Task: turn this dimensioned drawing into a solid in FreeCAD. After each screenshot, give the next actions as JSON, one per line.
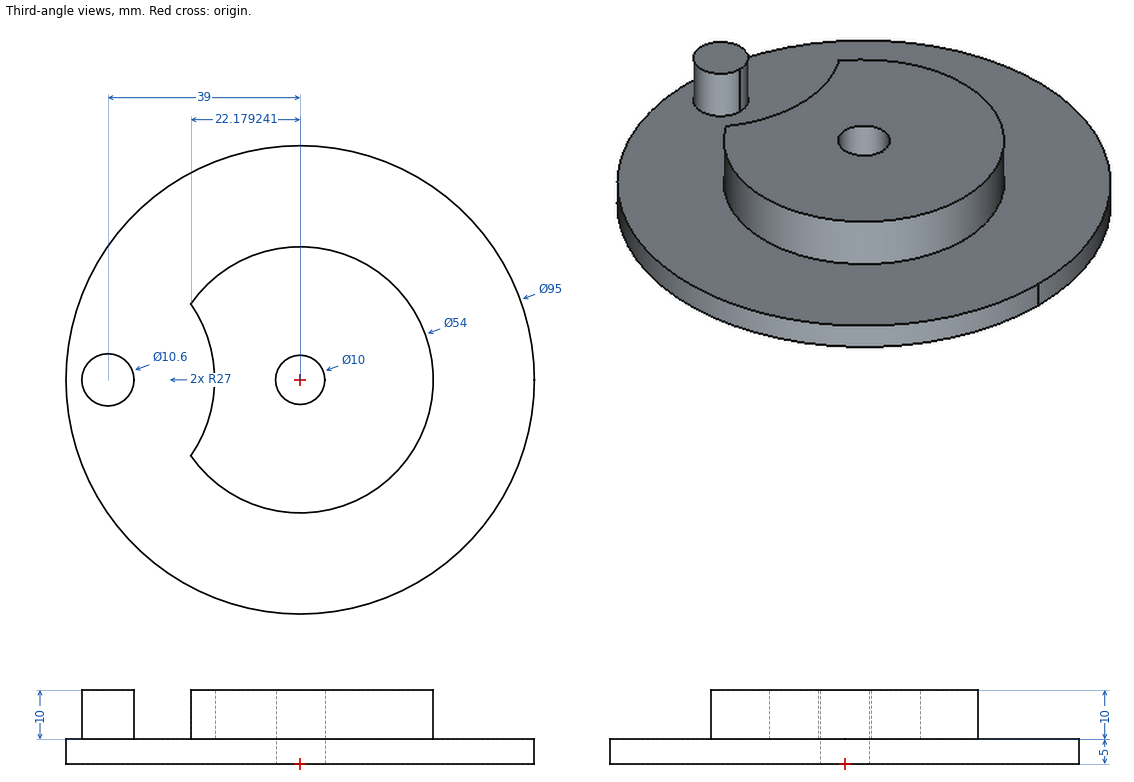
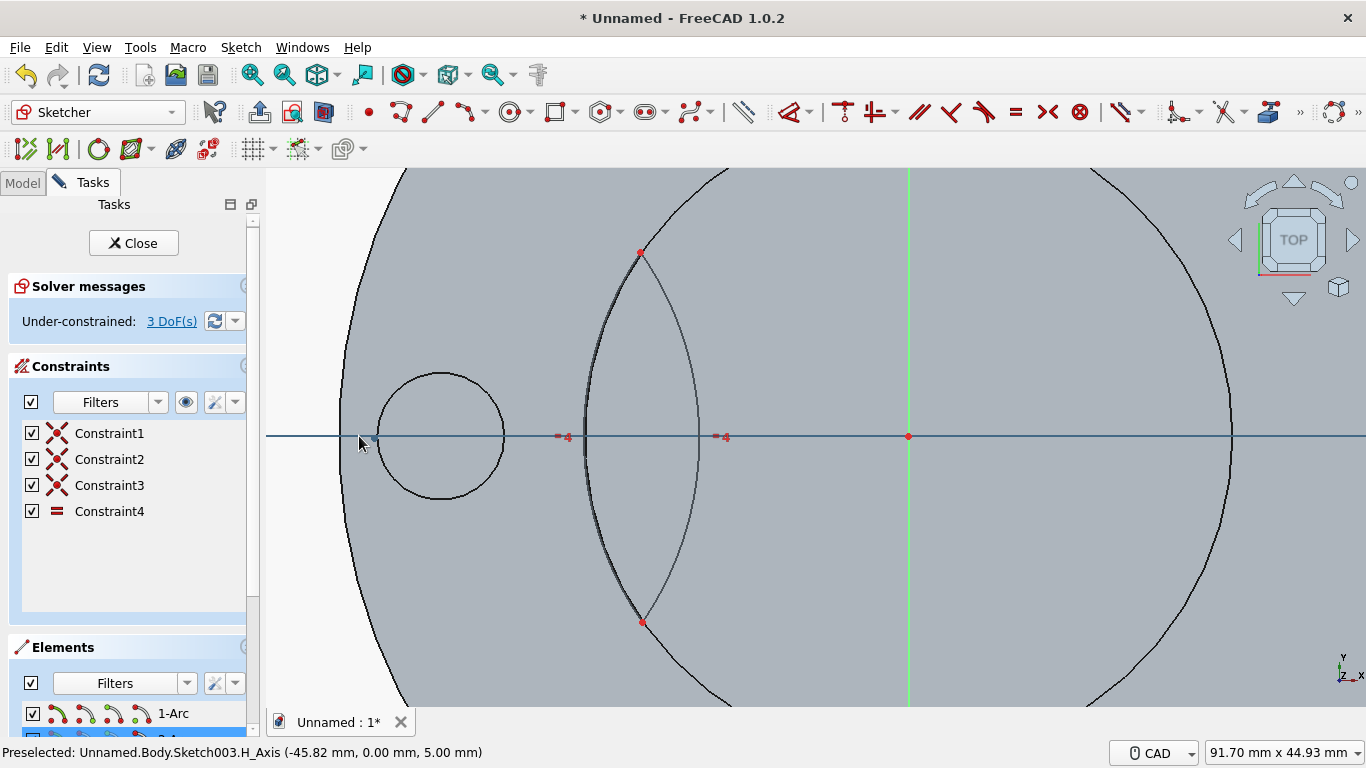
{"action": "key", "text": "c"}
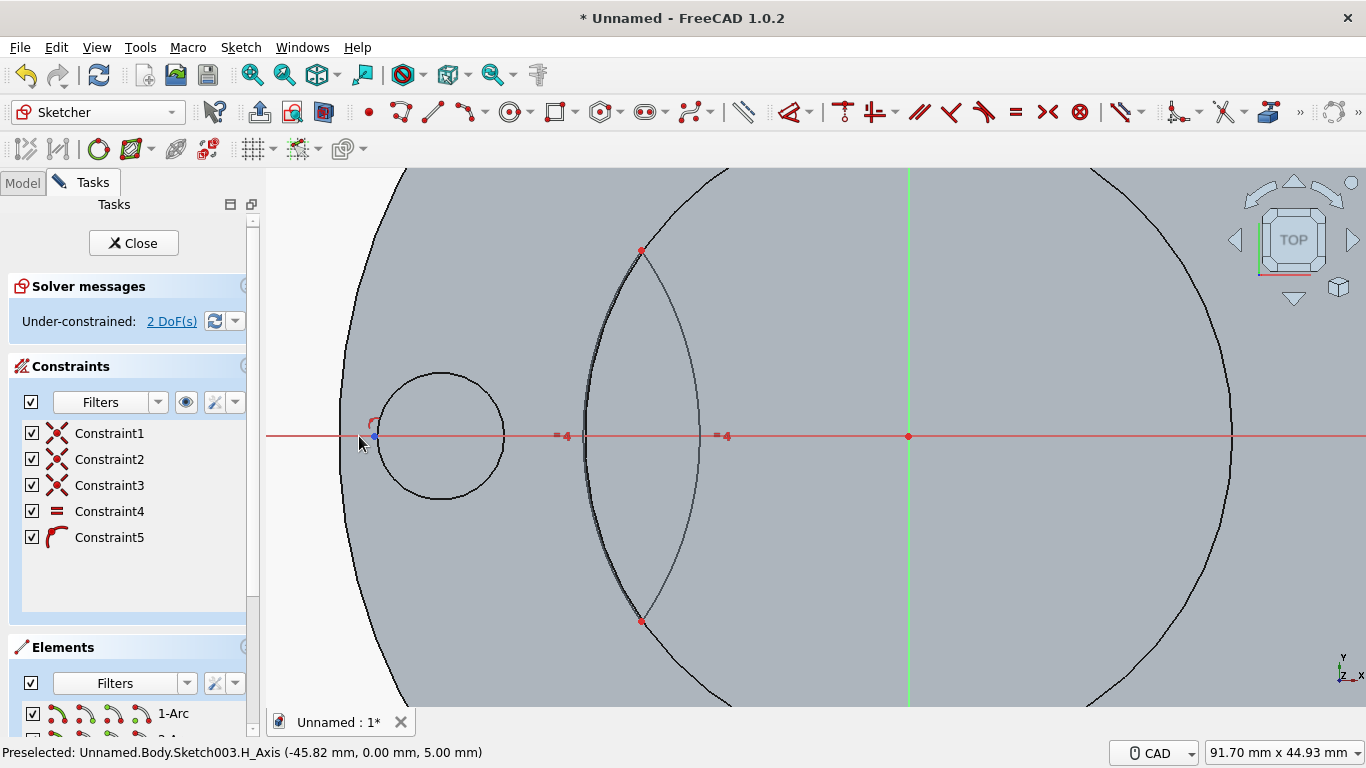
{"action": "key", "text": "d"}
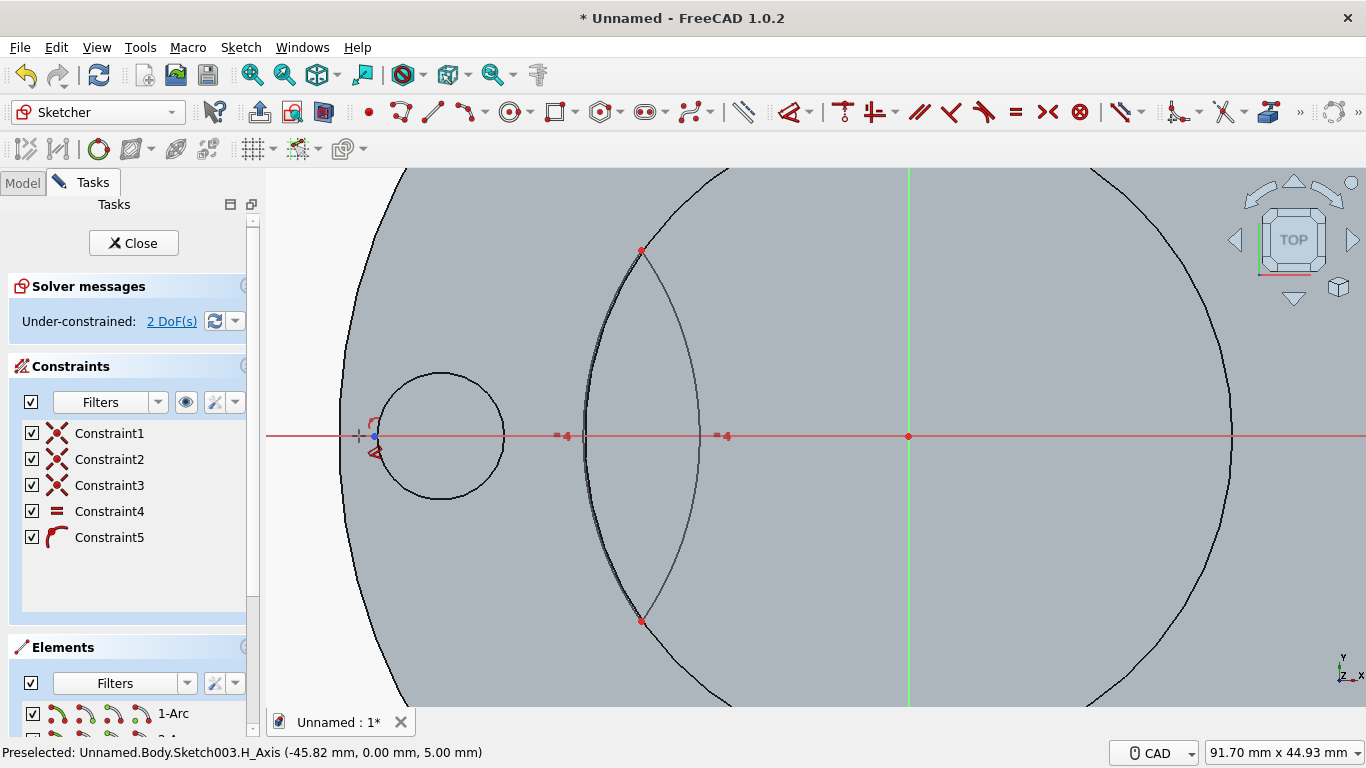
{"action": "left_click", "coordinate": [593, 358]}
{"action": "left_click", "coordinate": [562, 350]}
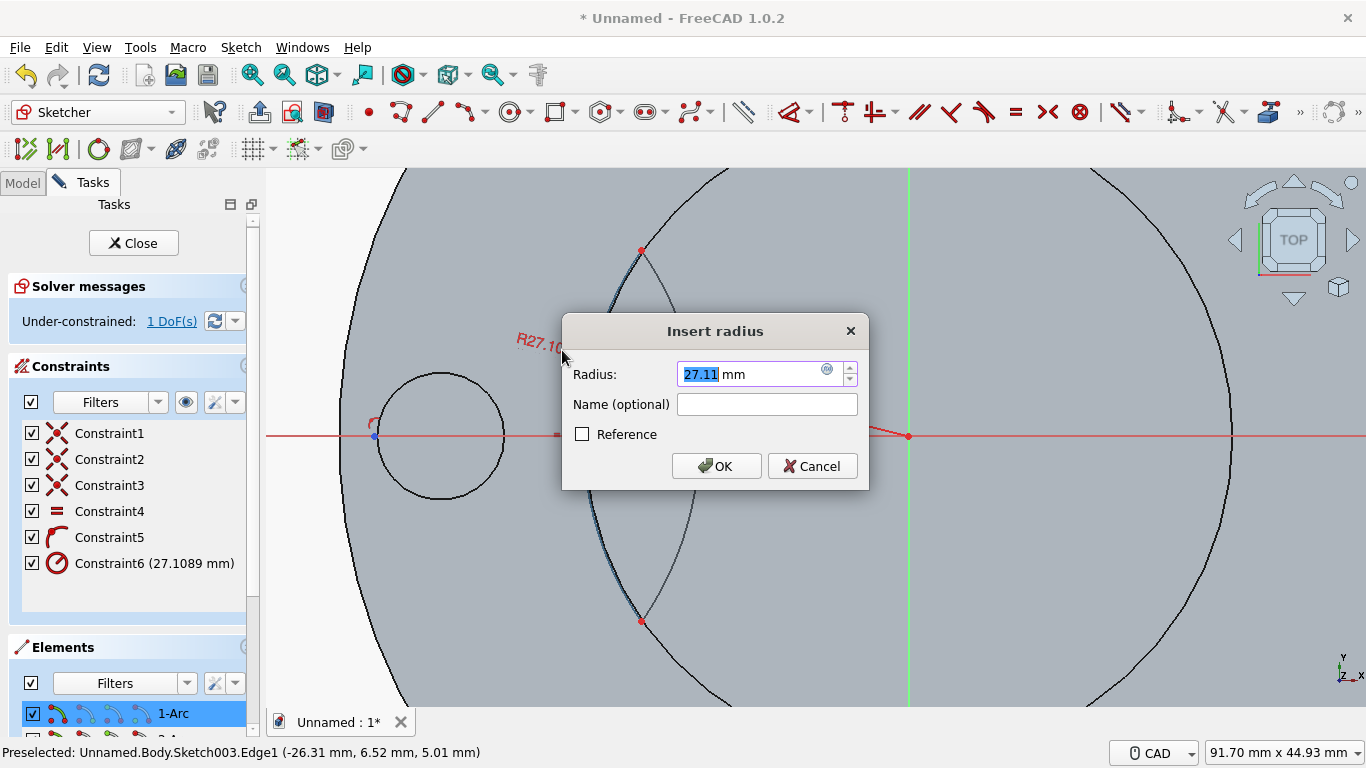
{"action": "type", "text": "27"}
{"action": "key", "text": "Return"}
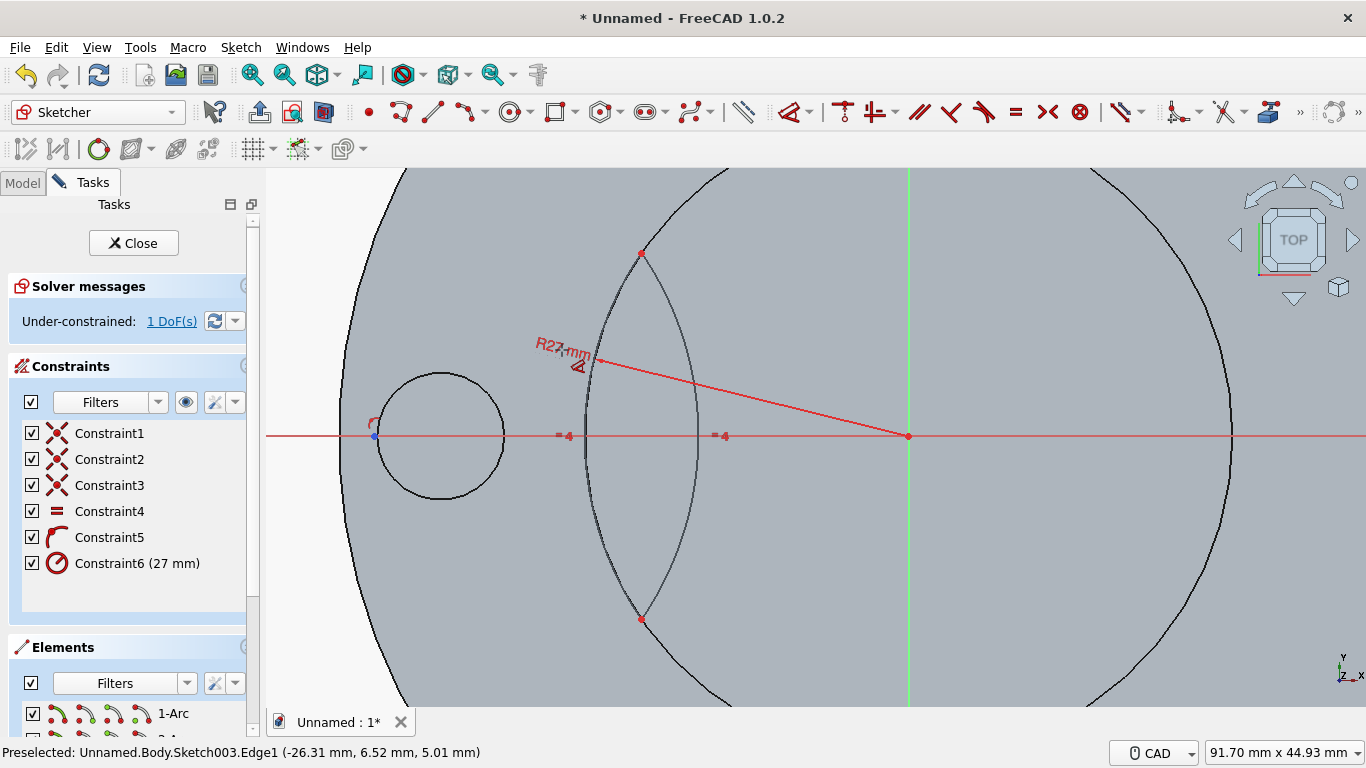
{"action": "left_click", "coordinate": [642, 253]}
{"action": "left_click", "coordinate": [775, 219]}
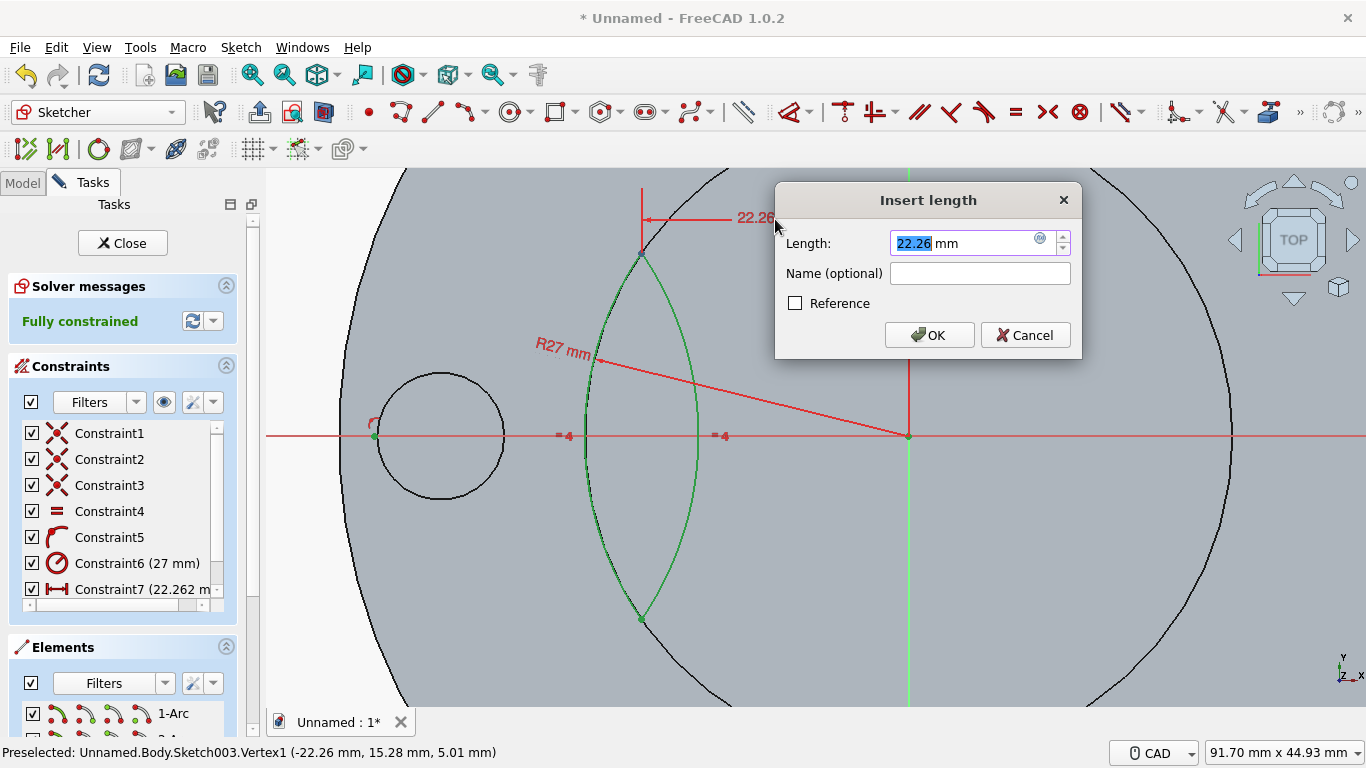
{"action": "type", "text": "22.179241"}
{"action": "key", "text": "Return"}
{"action": "key", "text": "Escape"}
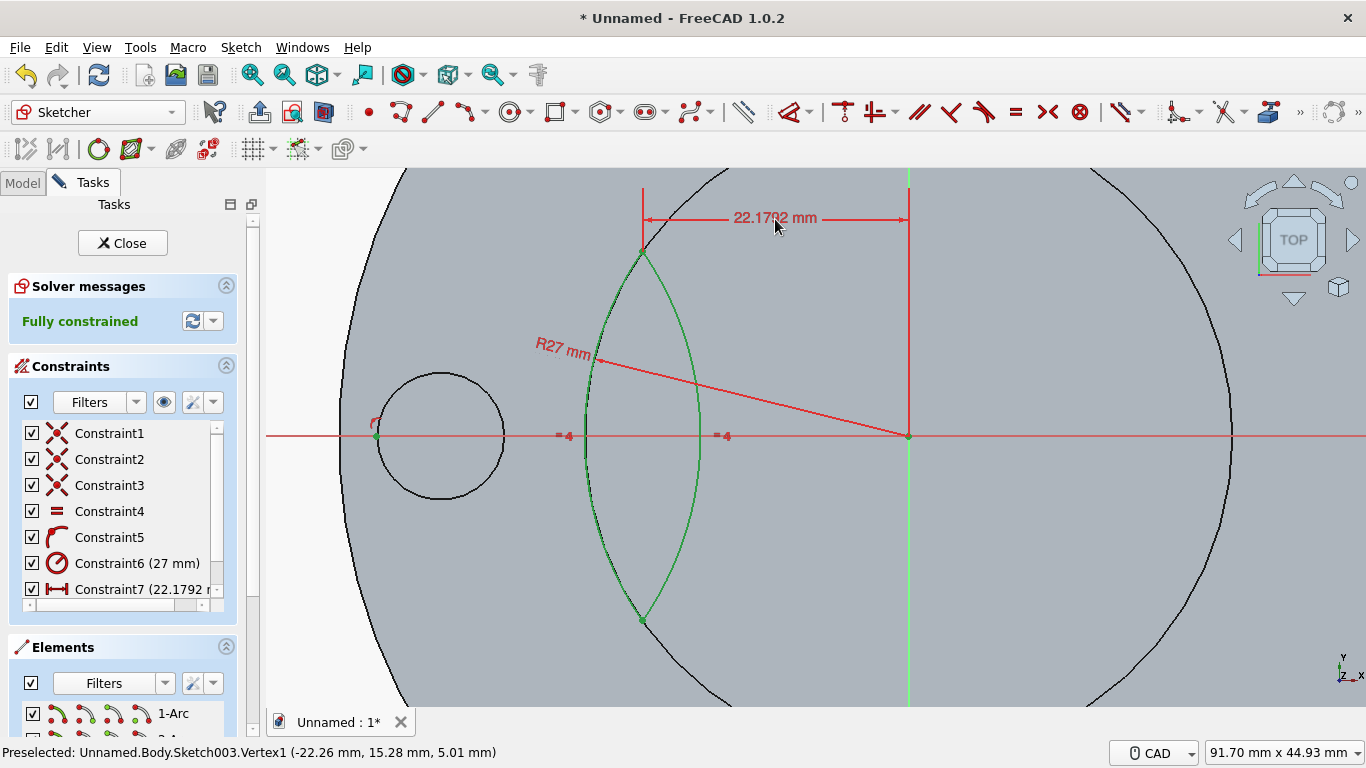
{"action": "left_click", "coordinate": [123, 243]}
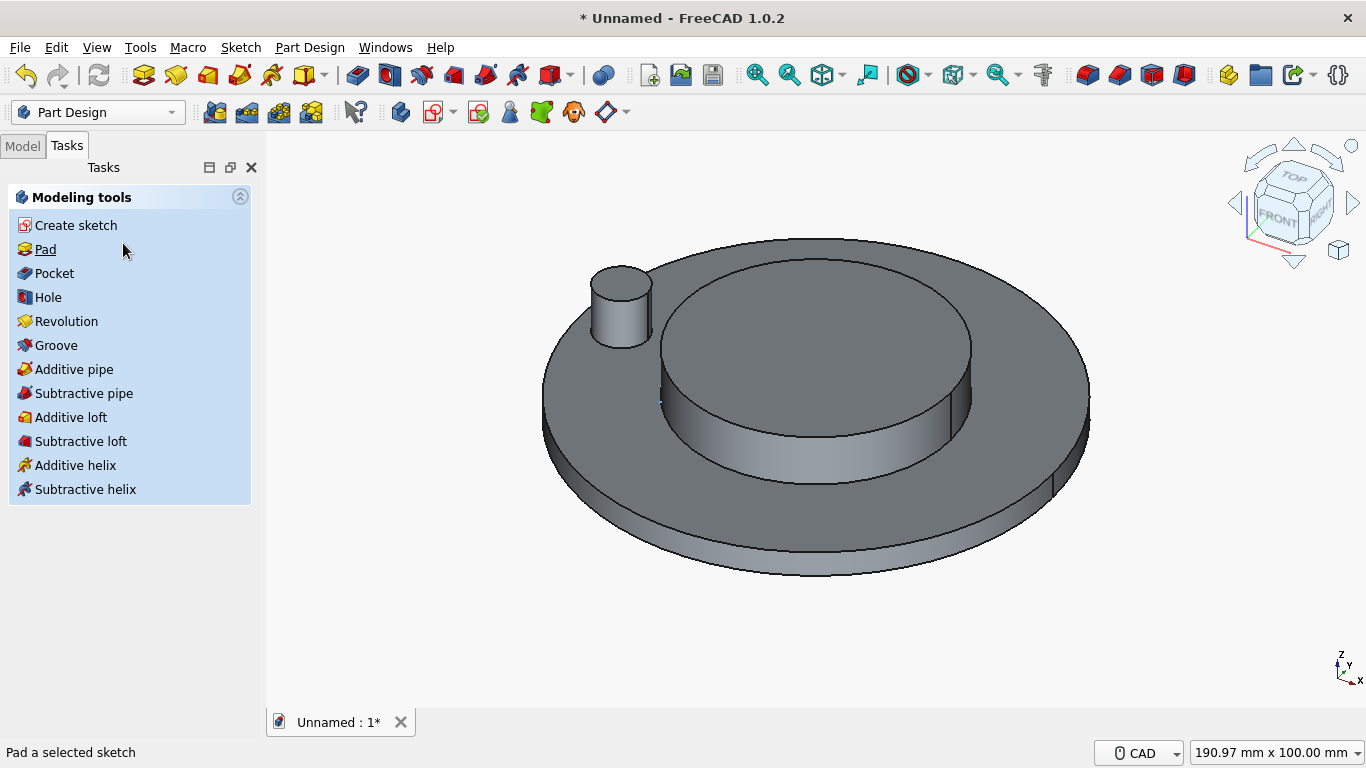
{"action": "left_click", "coordinate": [358, 76]}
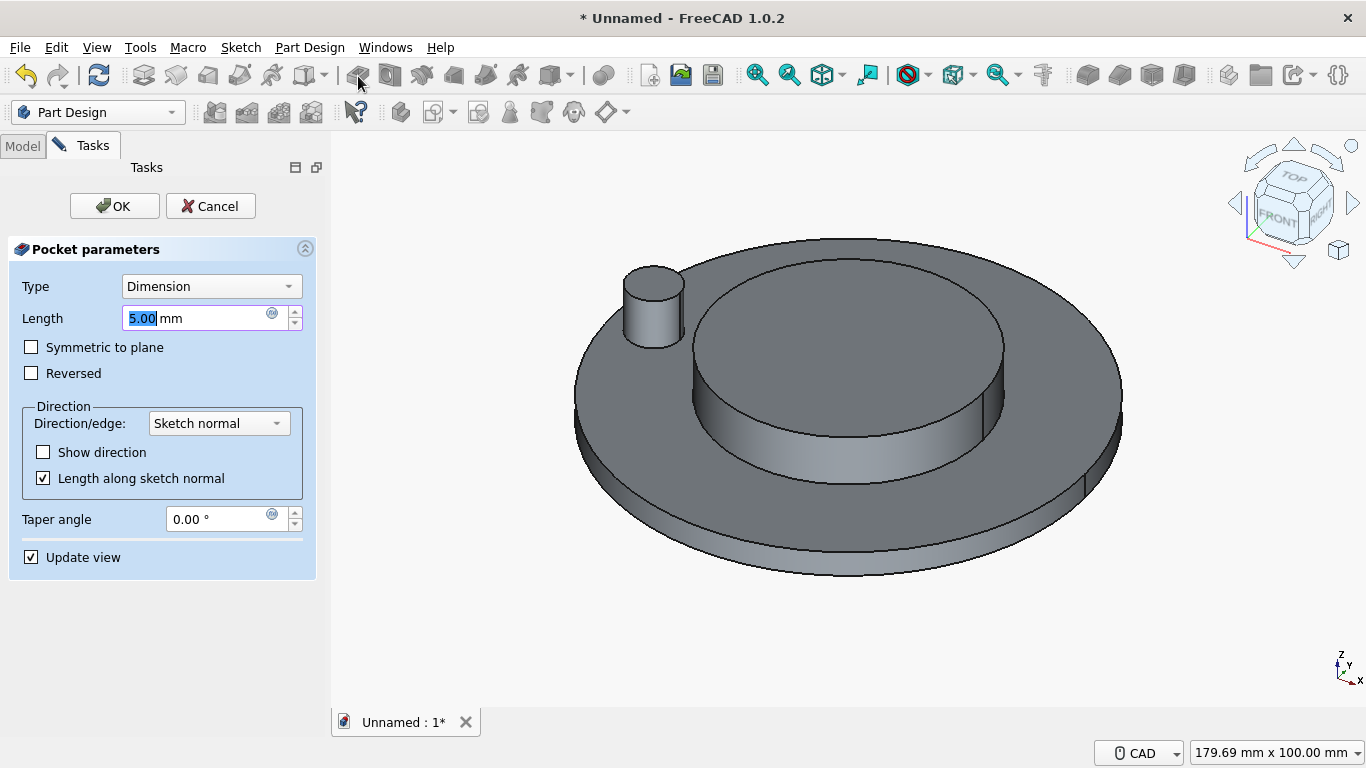
{"action": "type", "text": "10"}
{"action": "key", "text": "Tab"}